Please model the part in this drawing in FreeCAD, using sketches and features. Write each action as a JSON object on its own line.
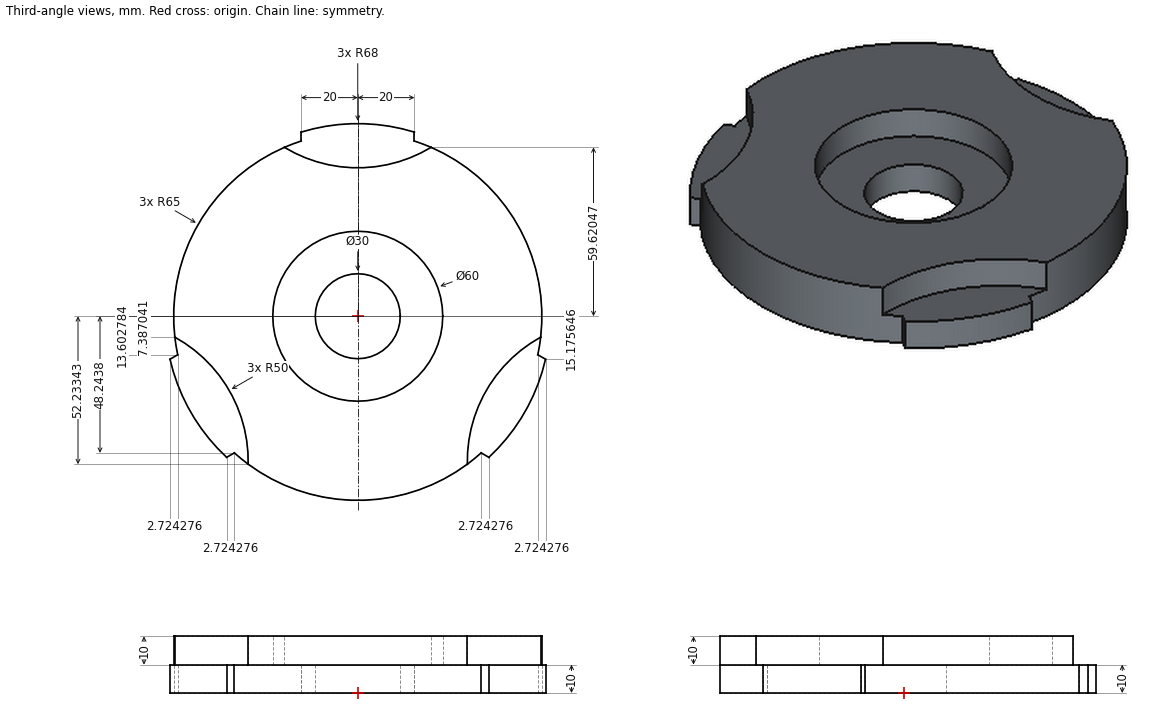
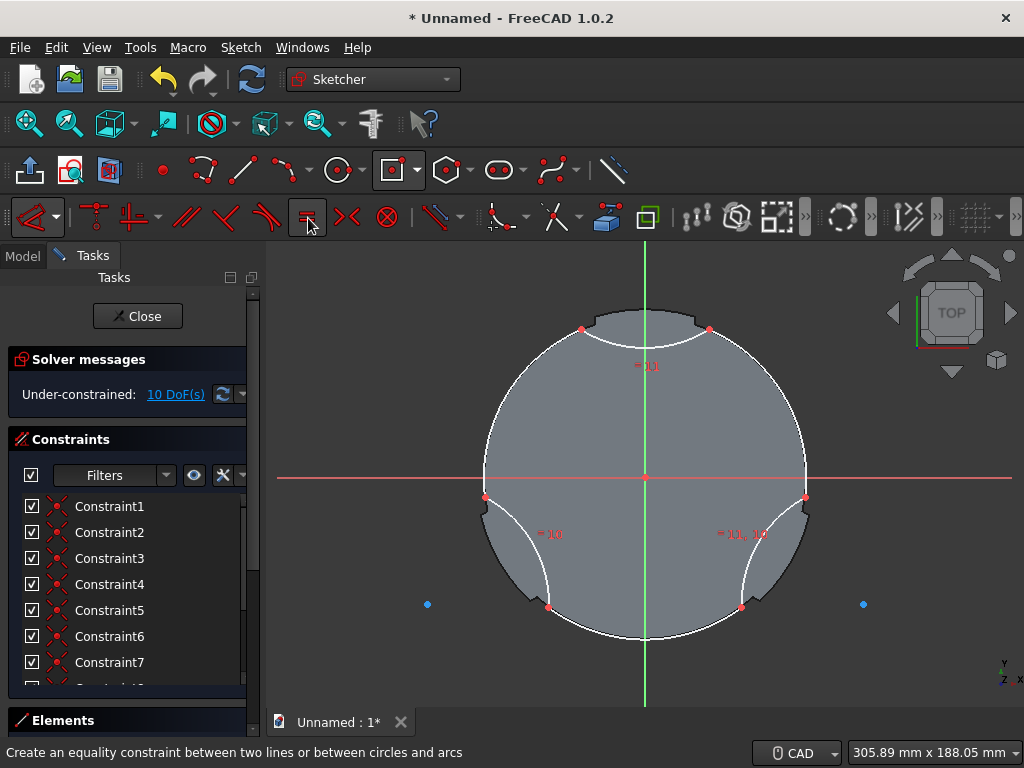
{"action": "left_click", "coordinate": [605, 634]}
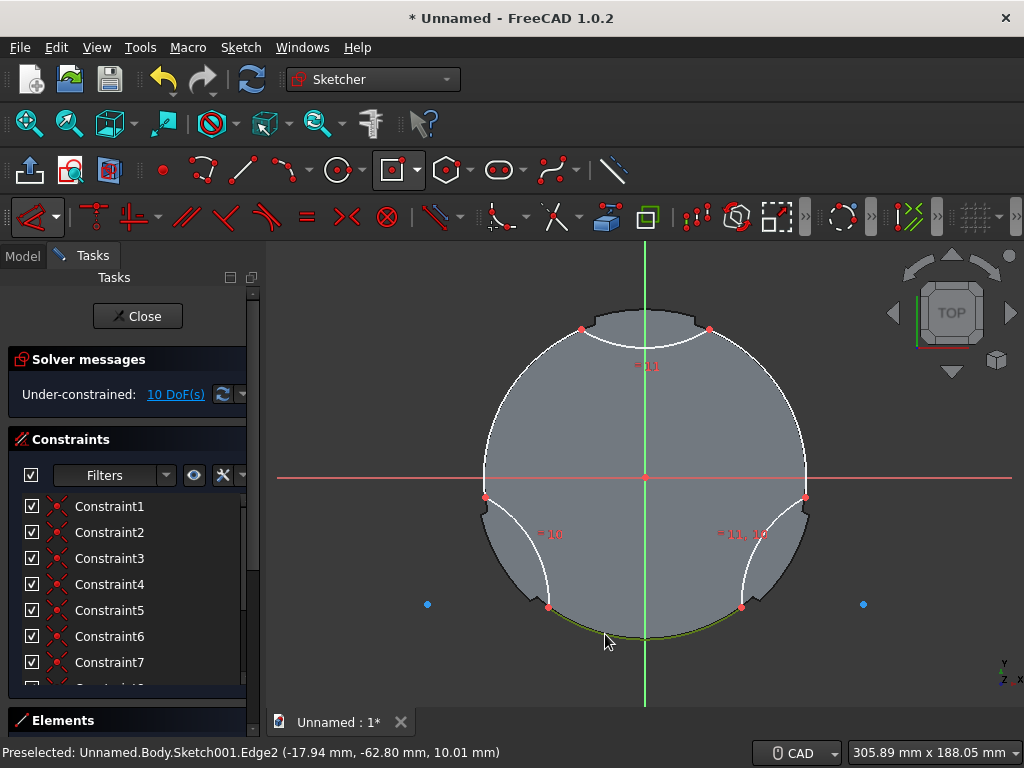
{"action": "left_click", "coordinate": [801, 436]}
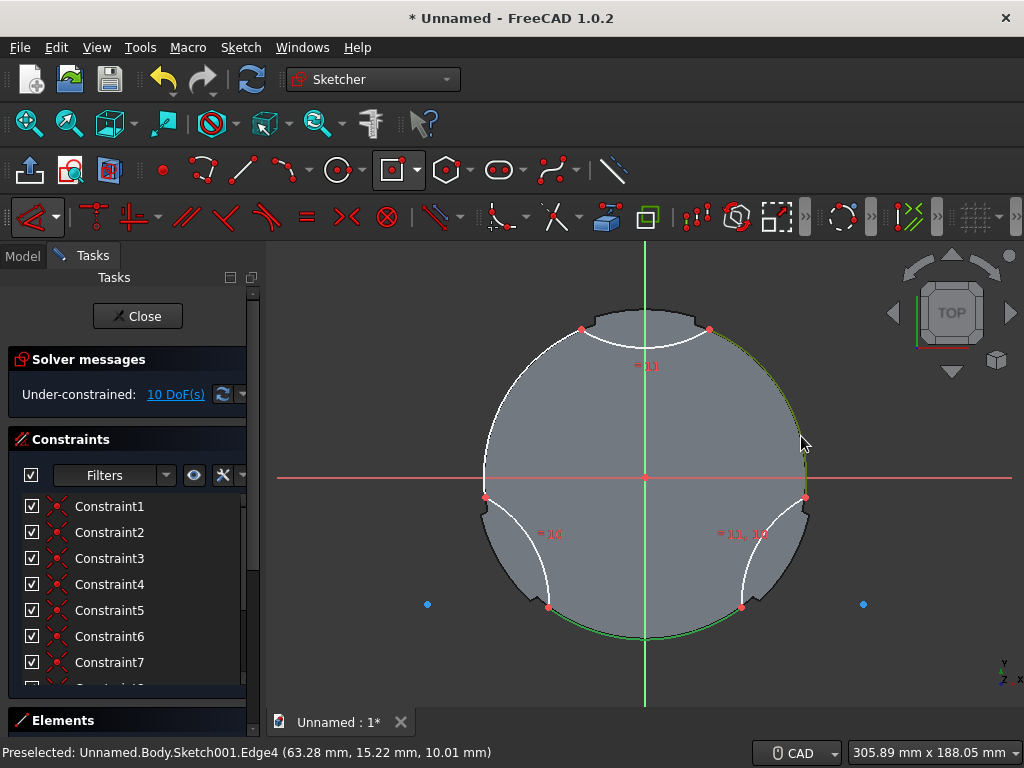
{"action": "left_click", "coordinate": [530, 365]}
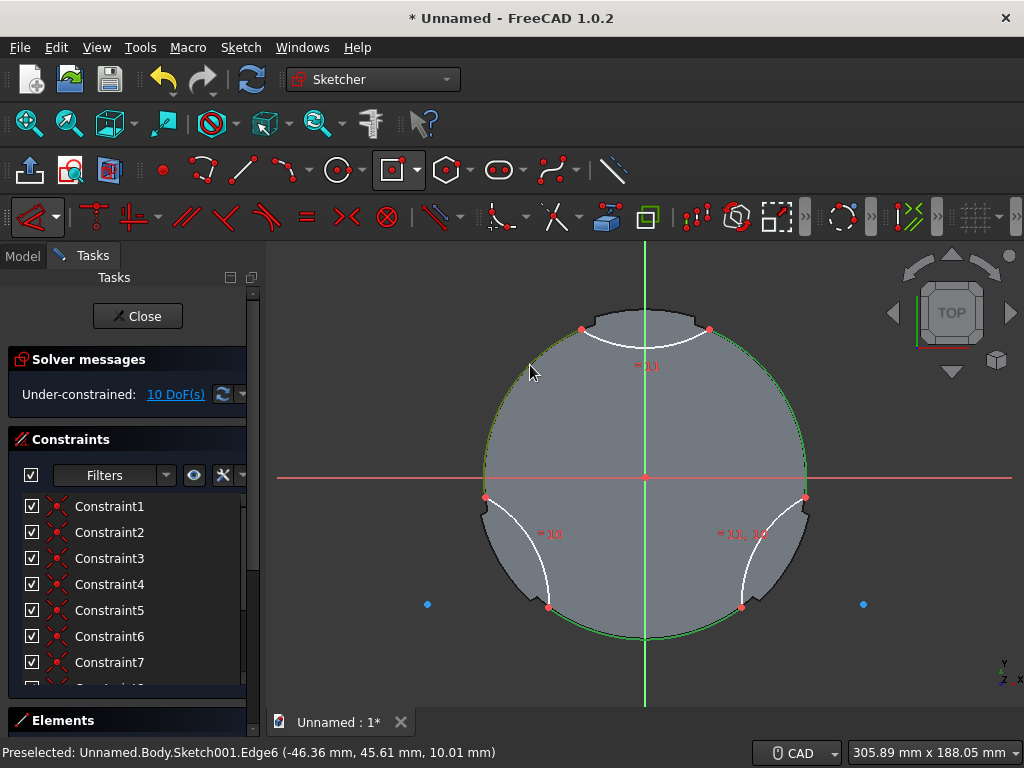
{"action": "left_click", "coordinate": [308, 218]}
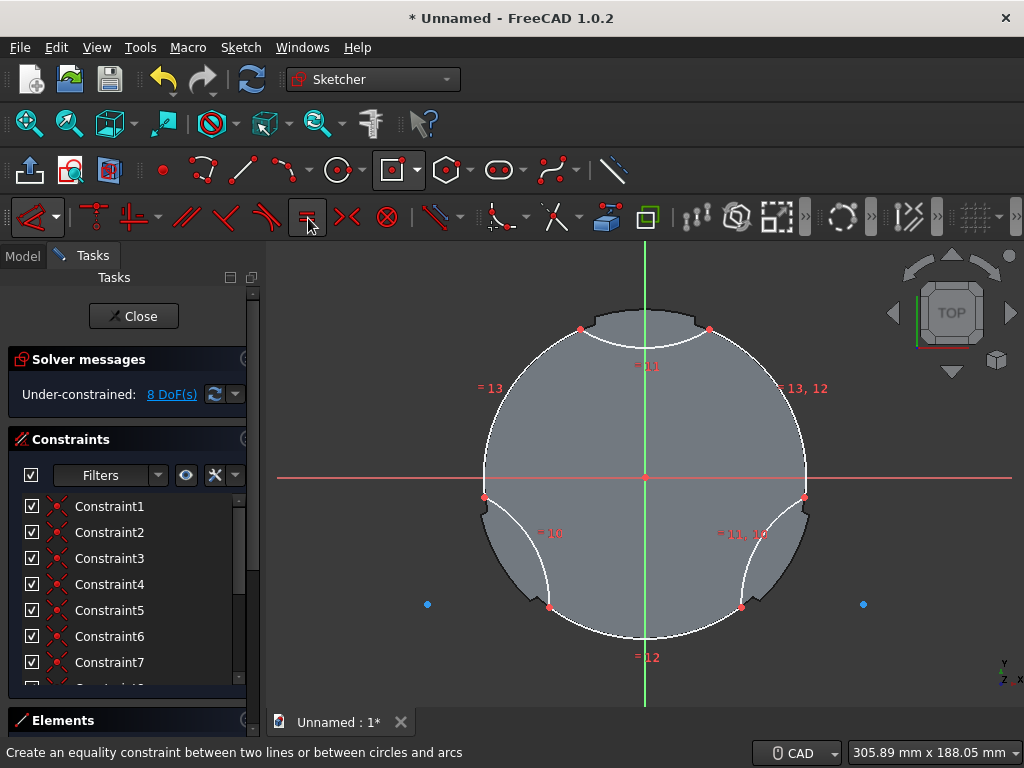
{"action": "scroll", "coordinate": [437, 558], "scroll_direction": "down", "scroll_amount": 2}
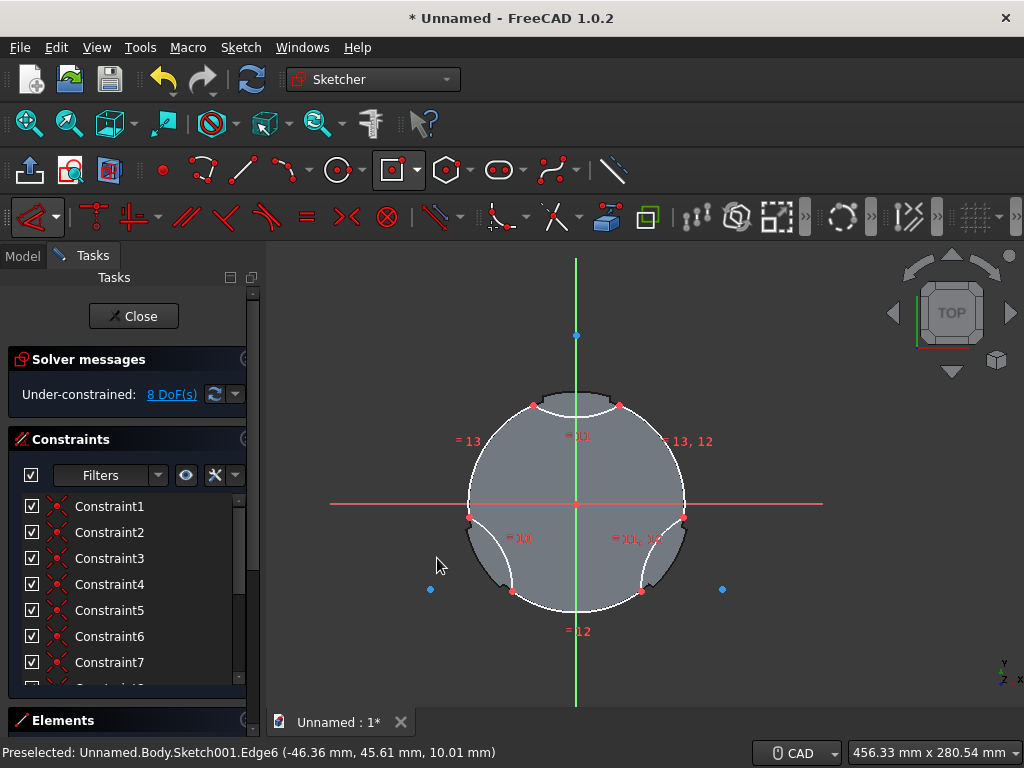
{"action": "left_click", "coordinate": [577, 336]}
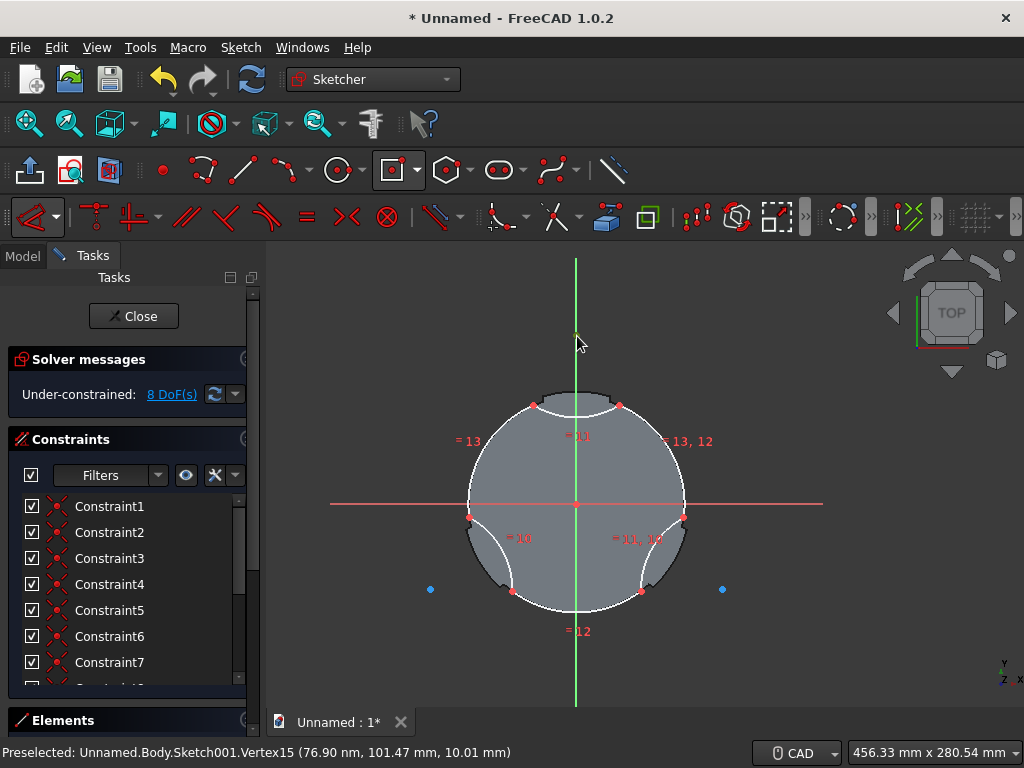
{"action": "left_click", "coordinate": [577, 650]}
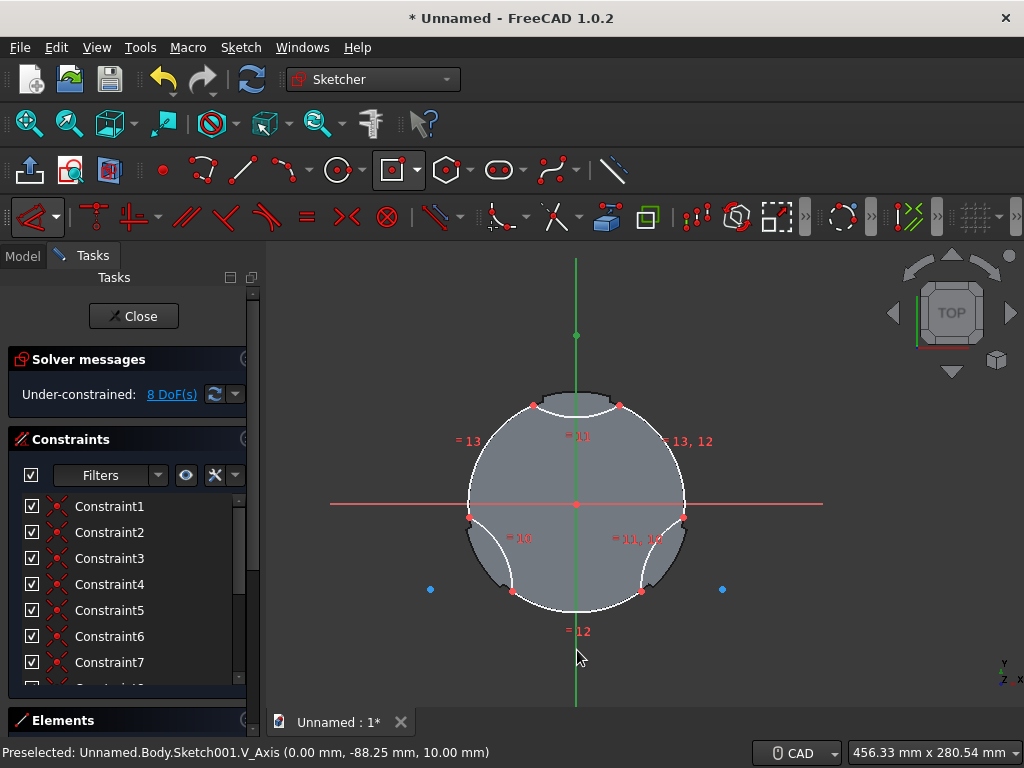
{"action": "left_click", "coordinate": [94, 218]}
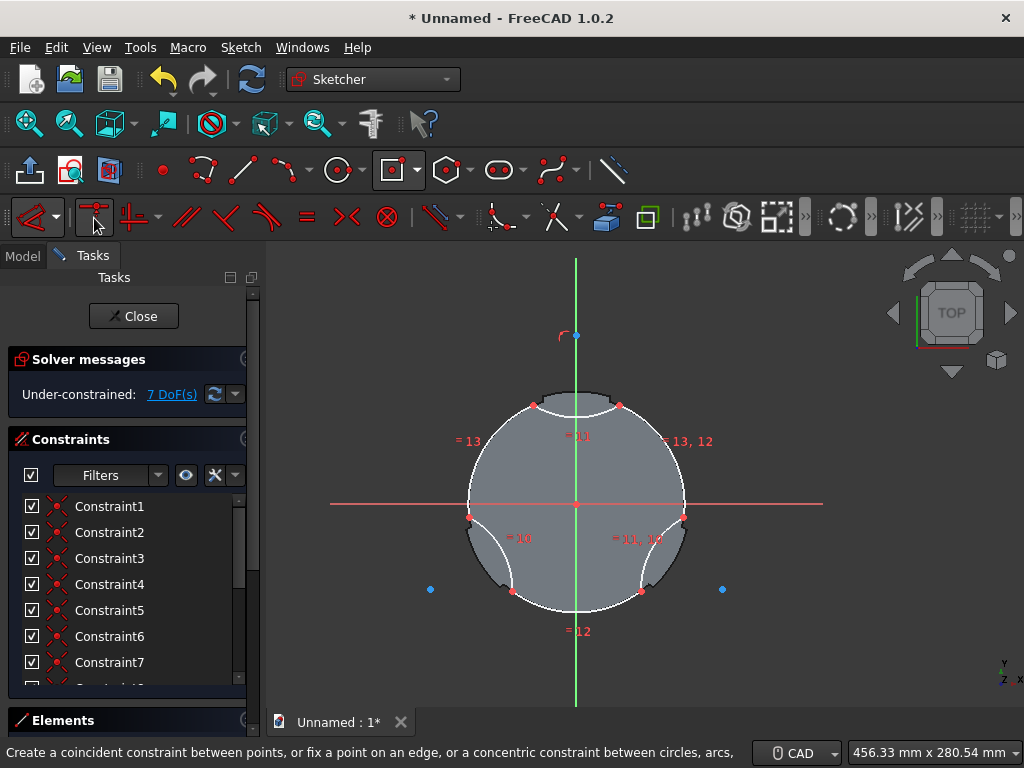
{"action": "left_click", "coordinate": [431, 590]}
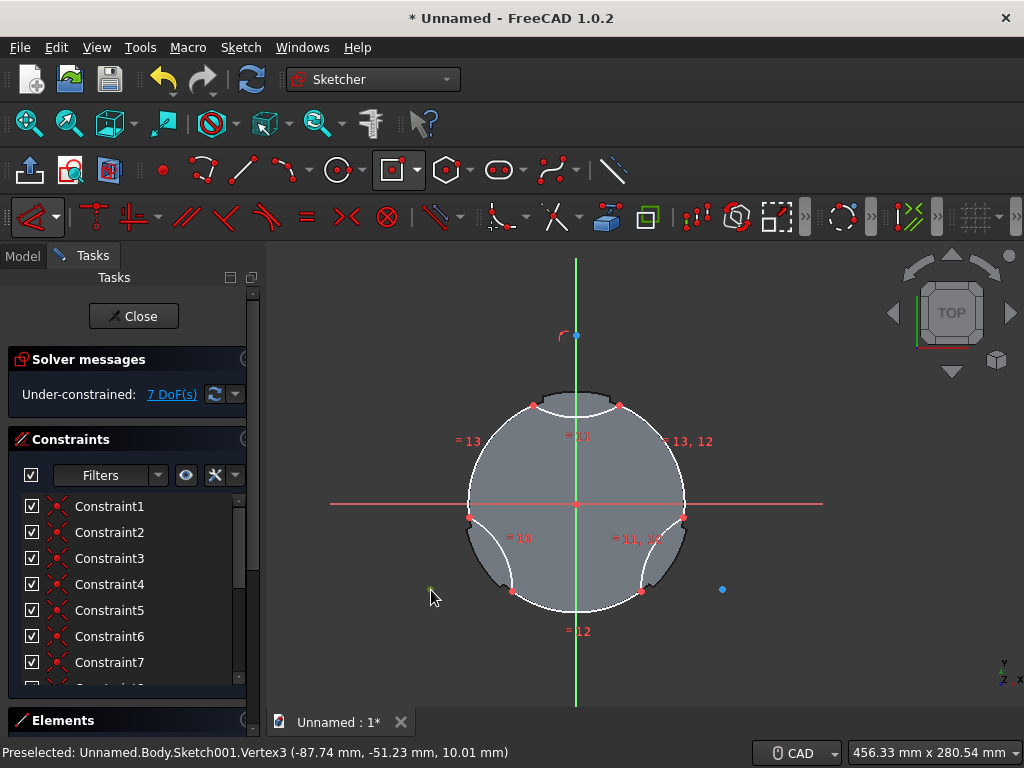
{"action": "left_click", "coordinate": [723, 590]}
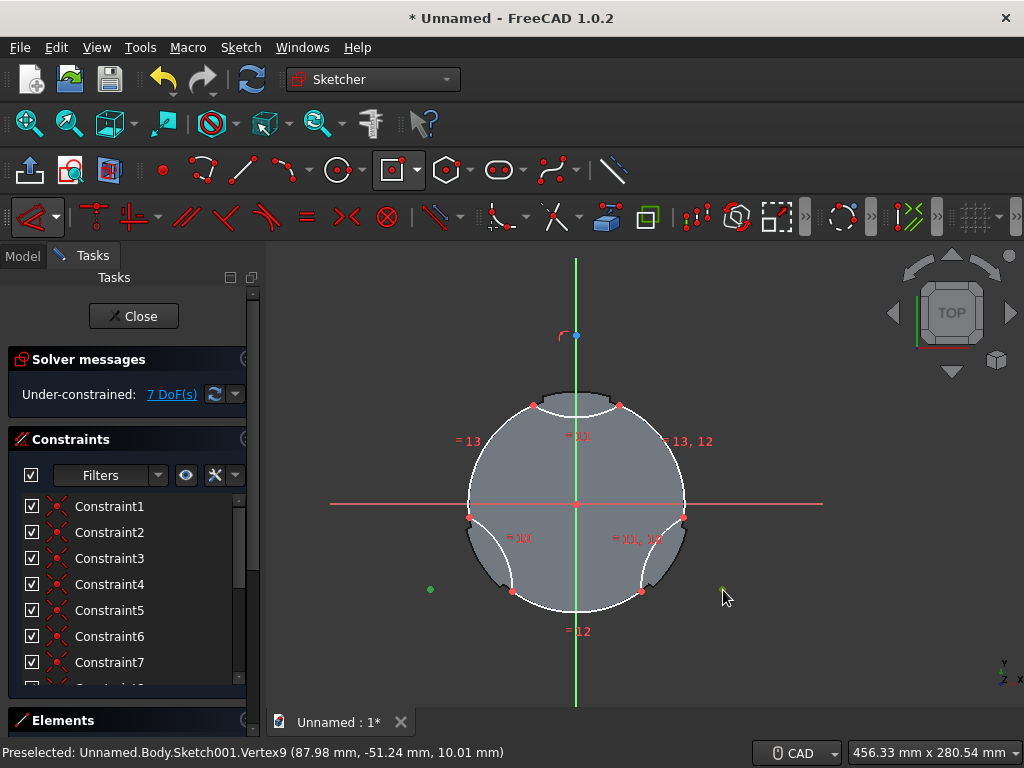
{"action": "left_click", "coordinate": [577, 650]}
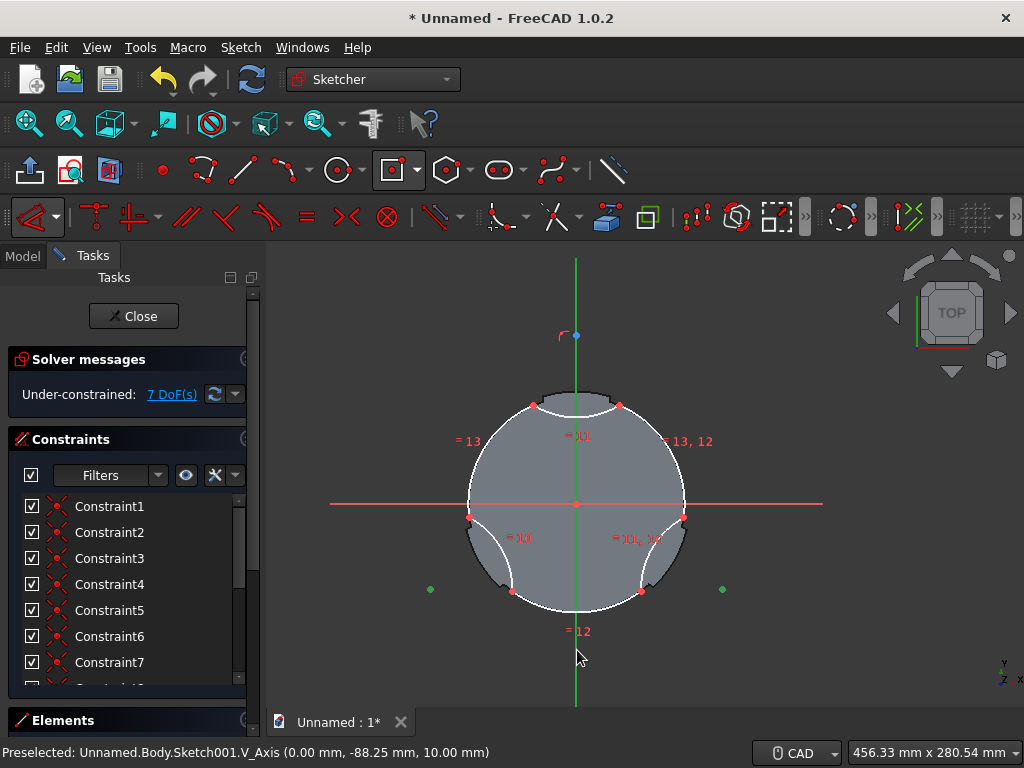
{"action": "key", "text": "s"}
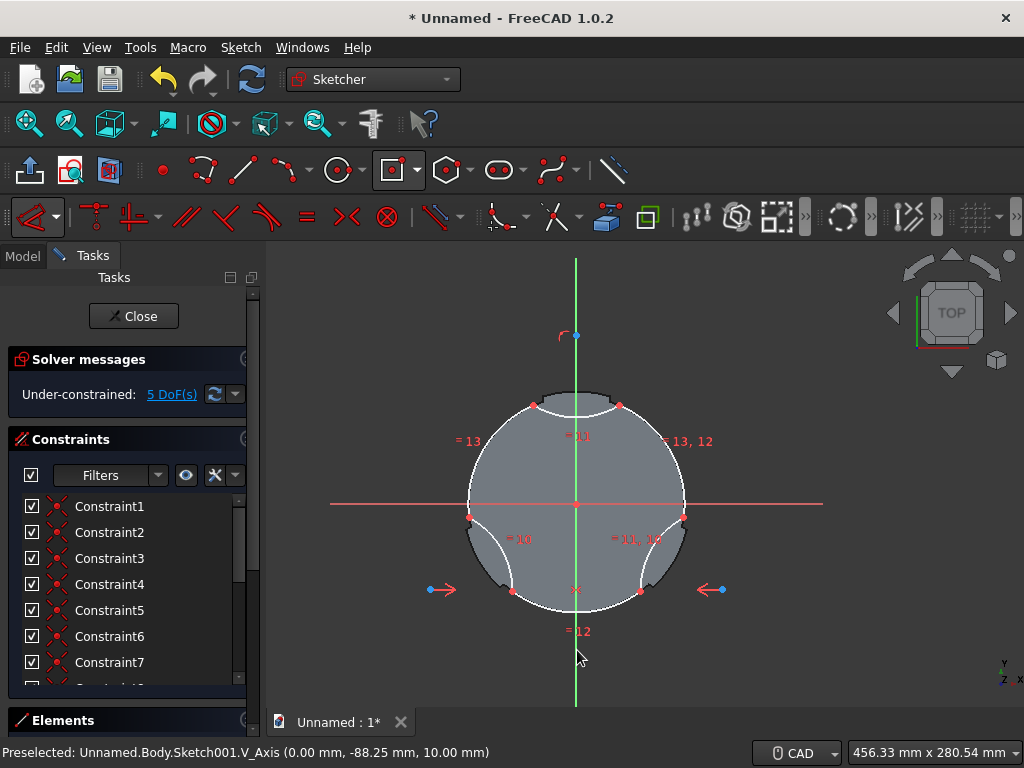
{"action": "left_click", "coordinate": [508, 565]}